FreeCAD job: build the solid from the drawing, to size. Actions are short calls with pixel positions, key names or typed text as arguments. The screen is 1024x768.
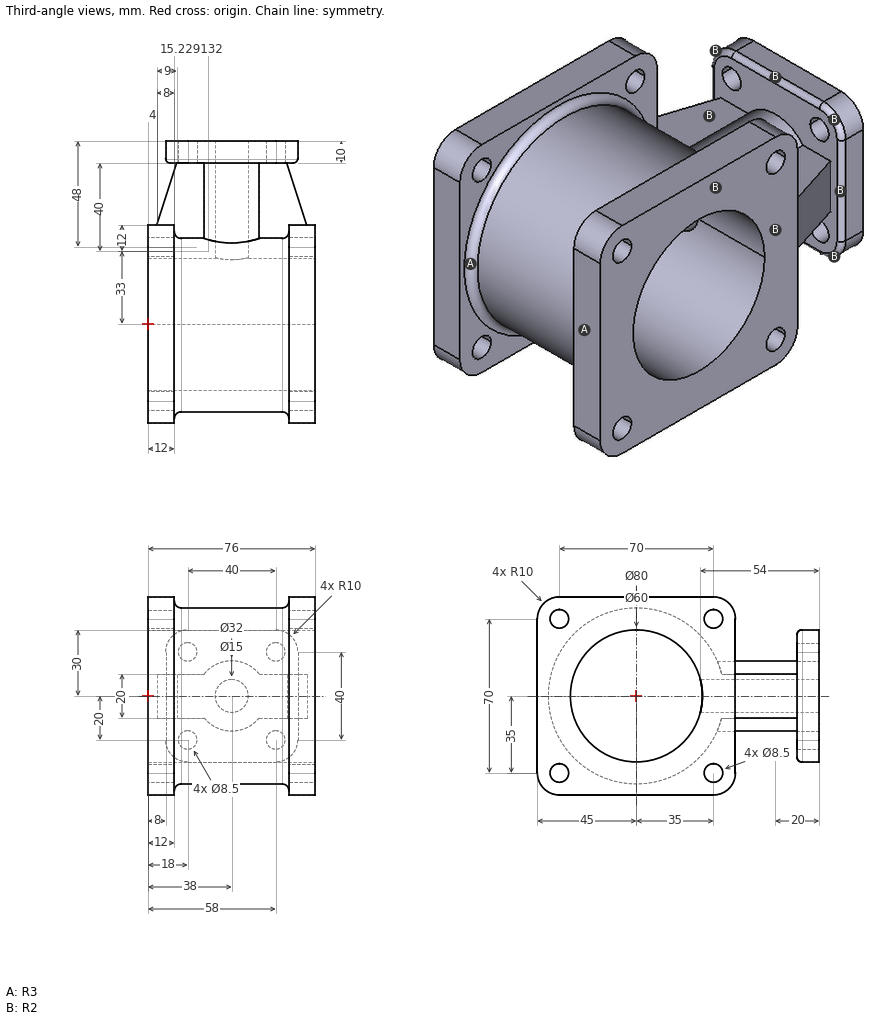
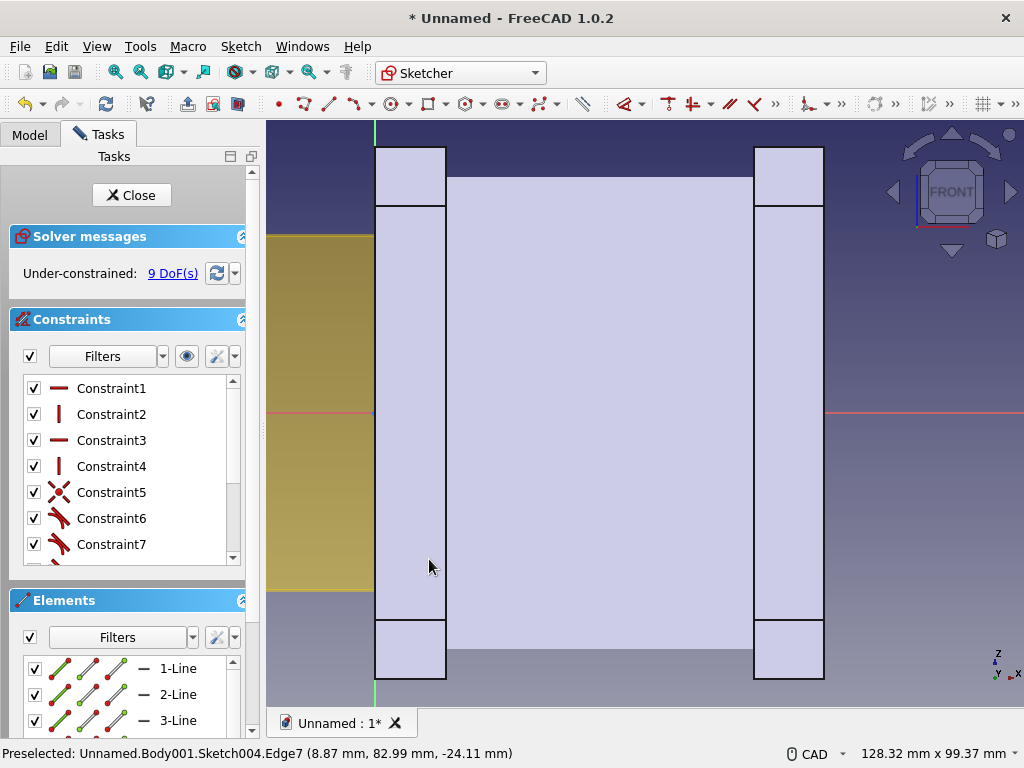
click(423, 461)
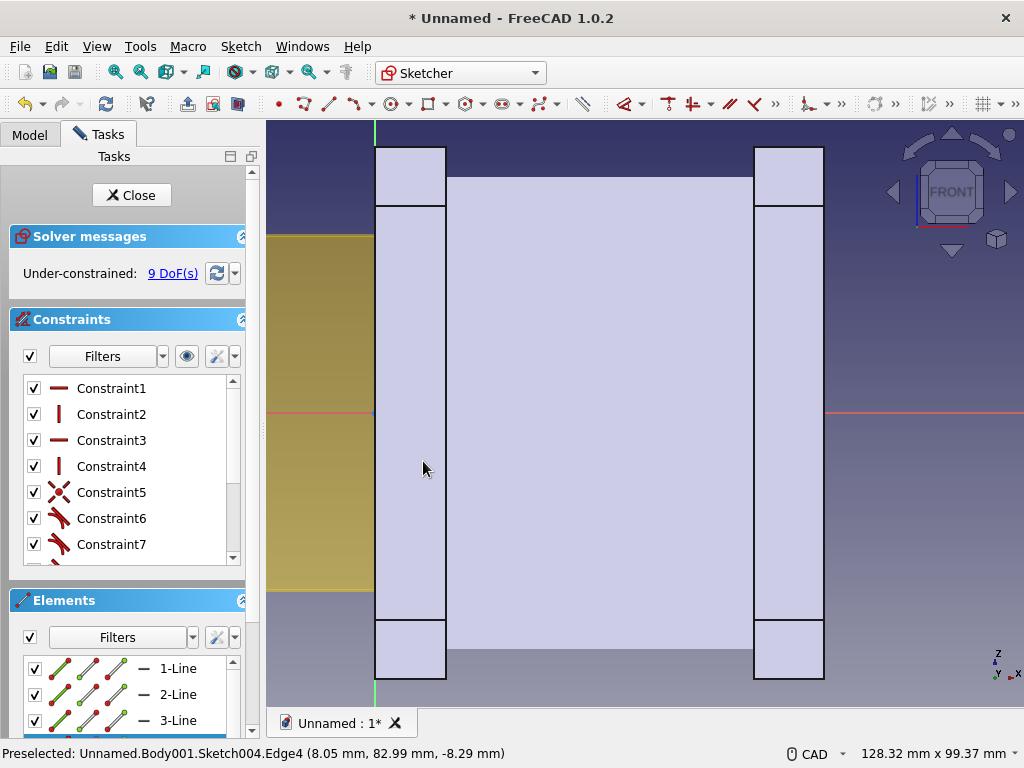
click(455, 243)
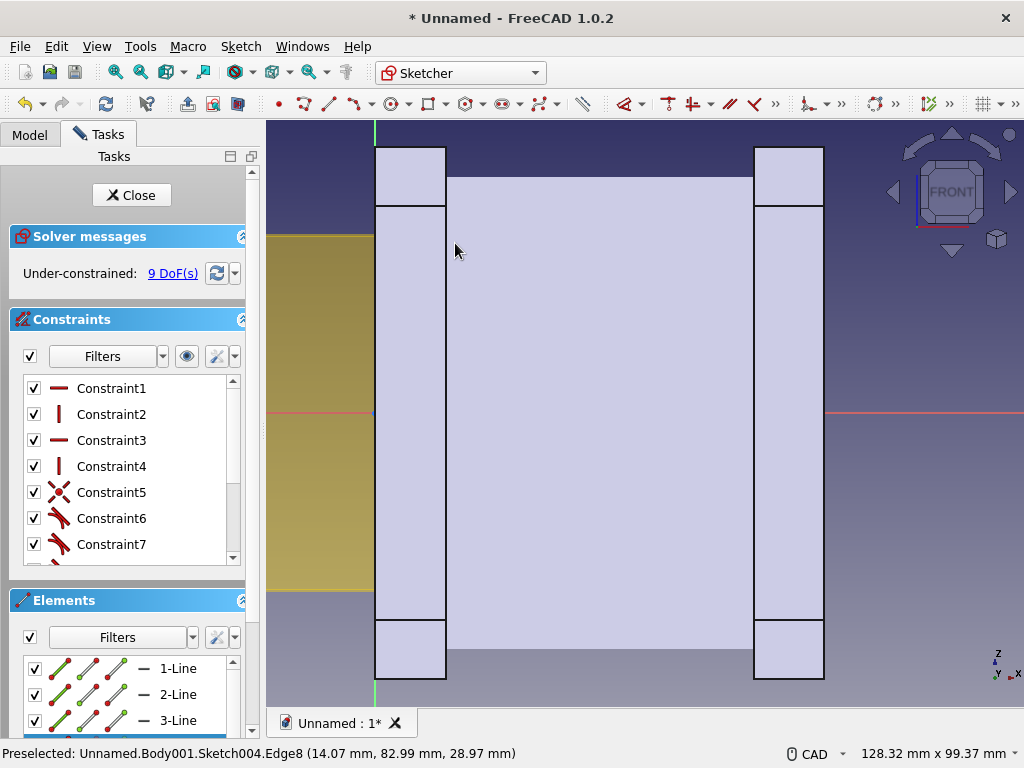
key(t)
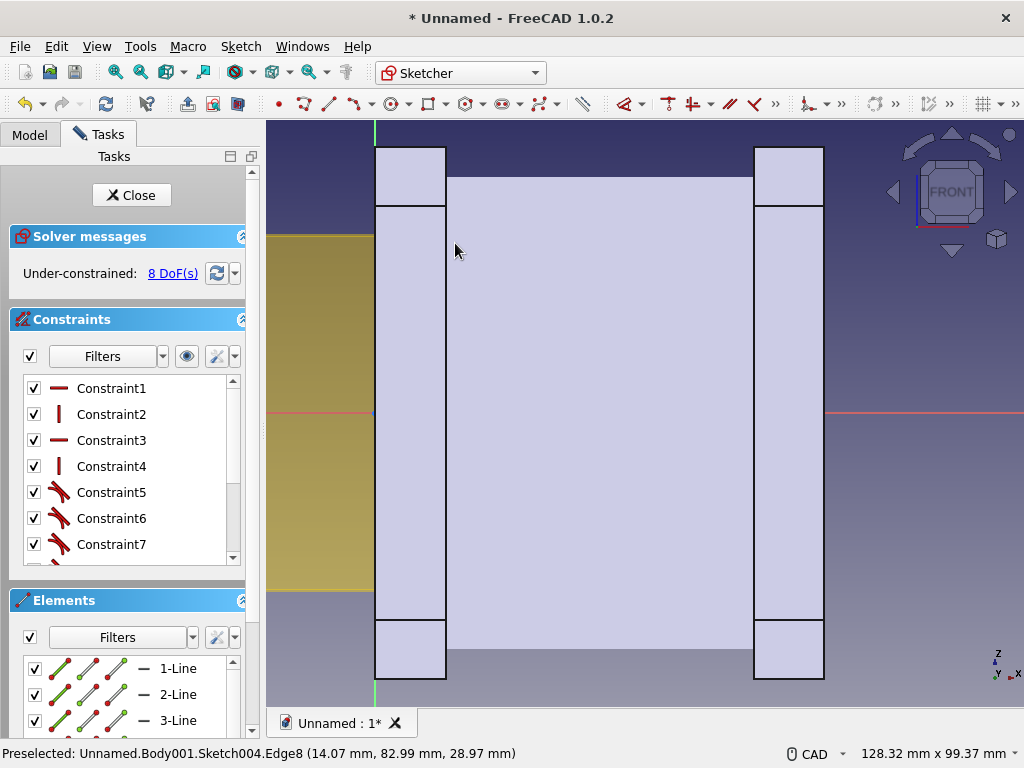
click(771, 269)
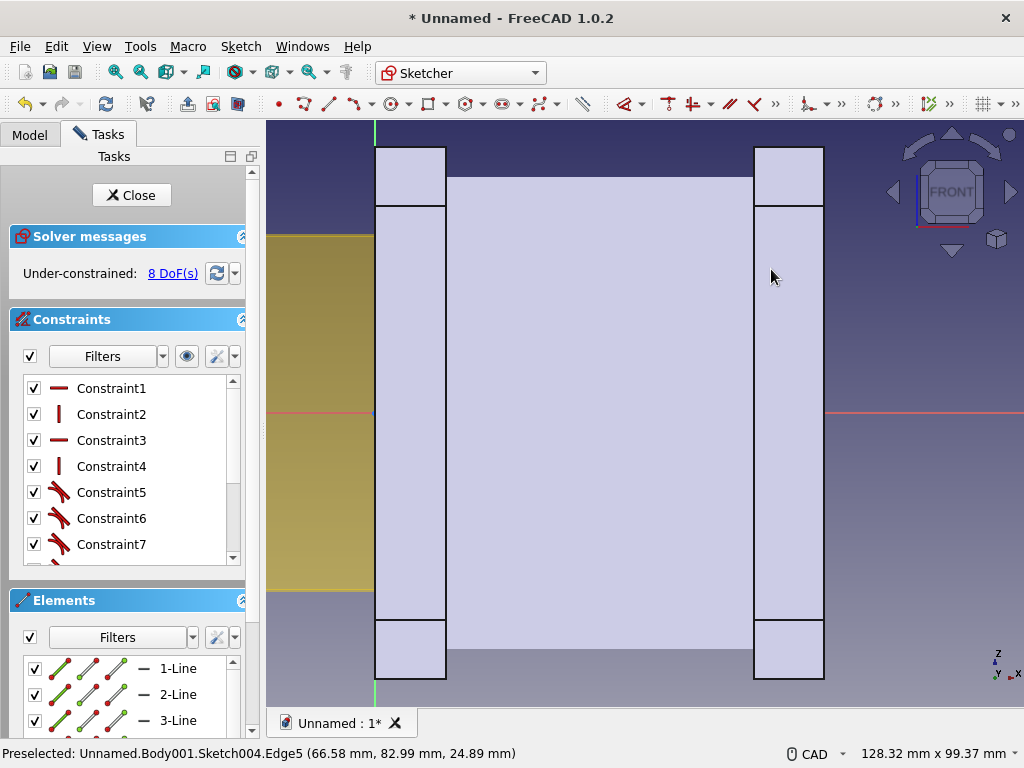
click(745, 585)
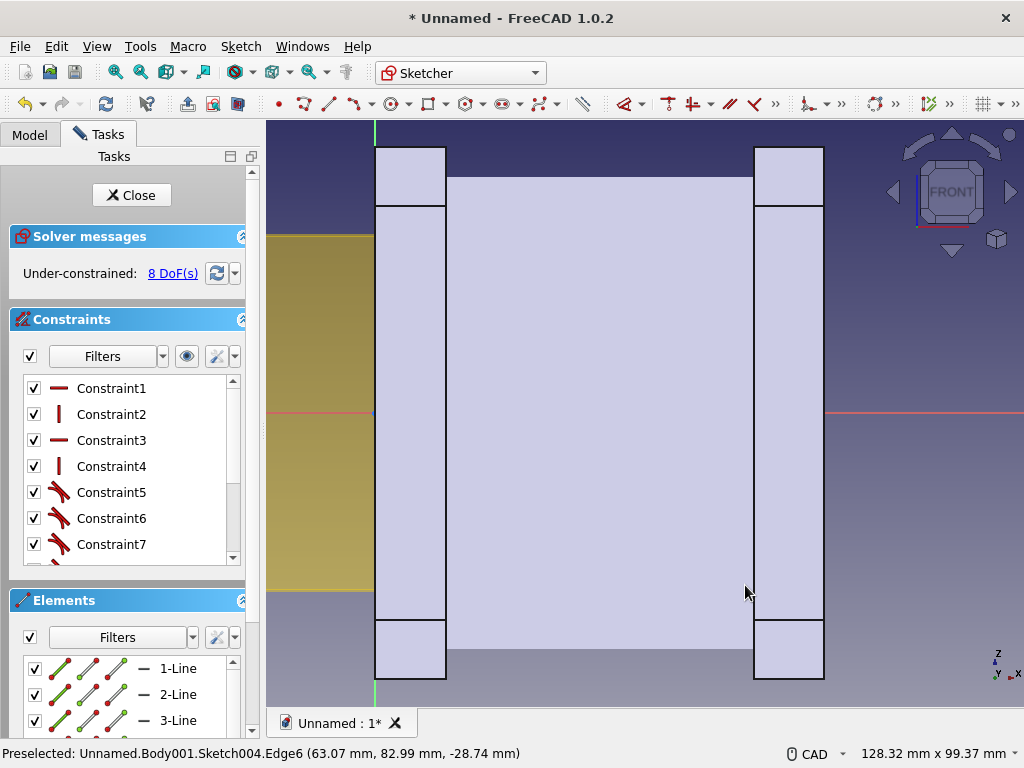
click(429, 559)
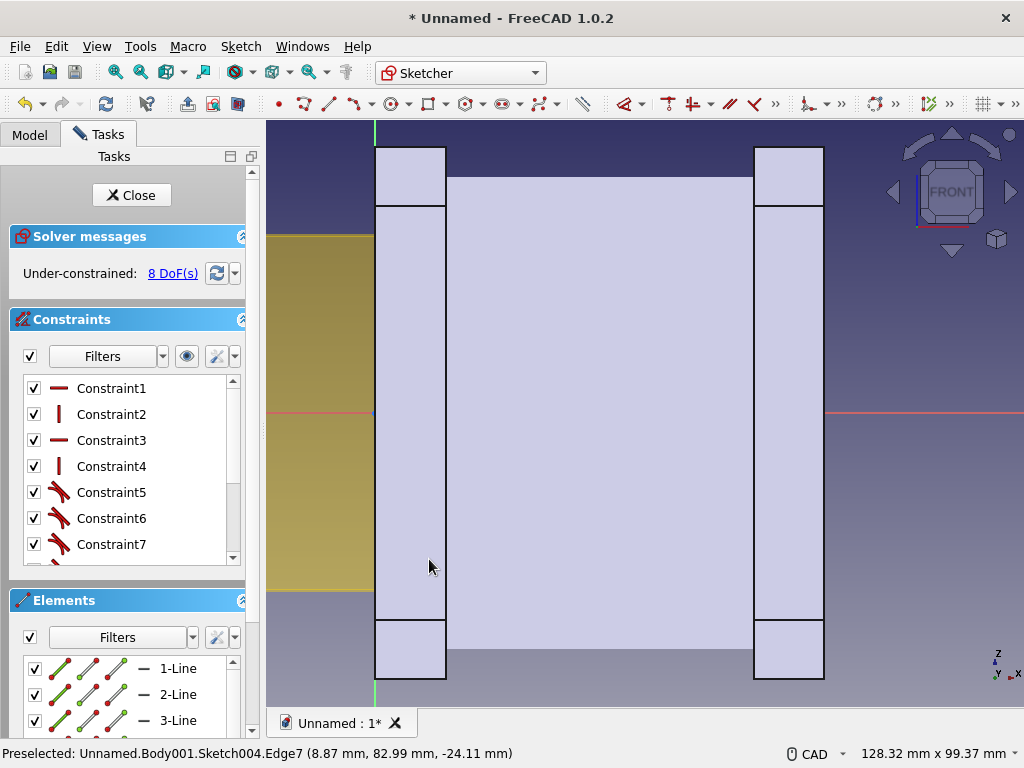
click(455, 243)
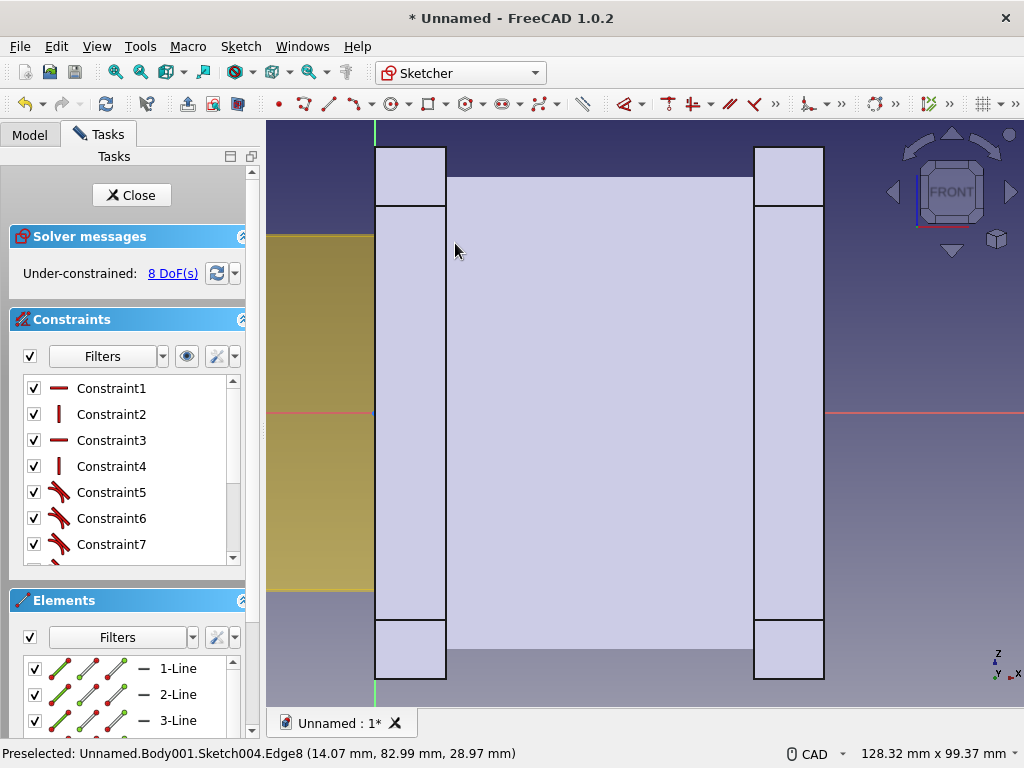
key(e)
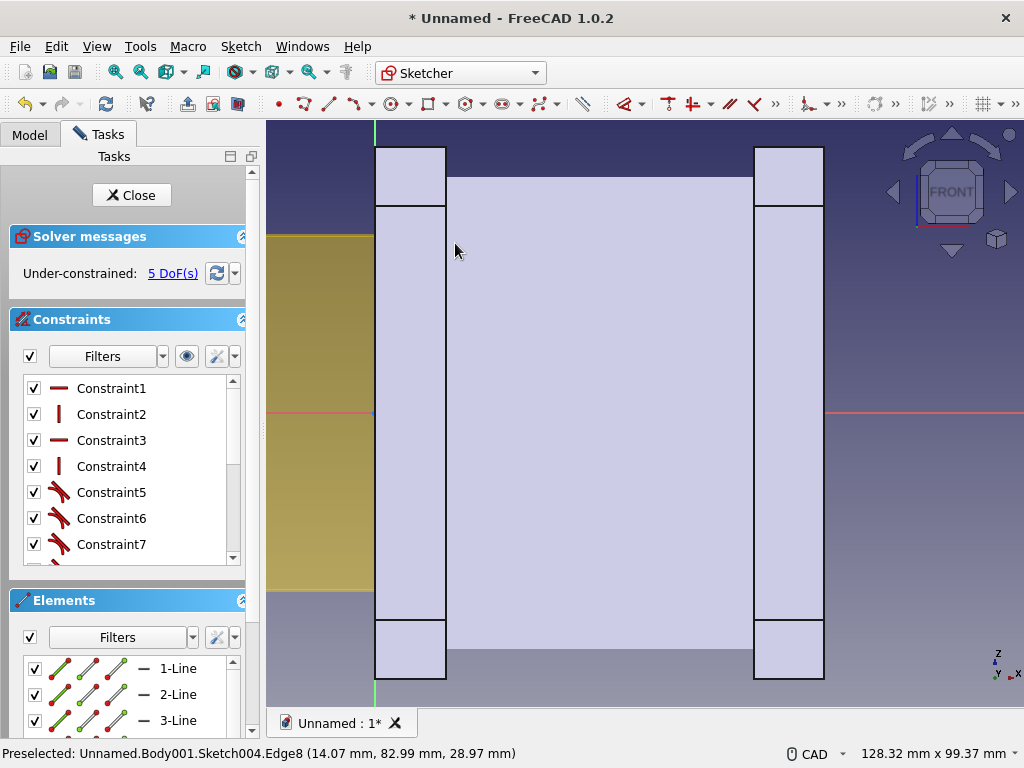
key(d)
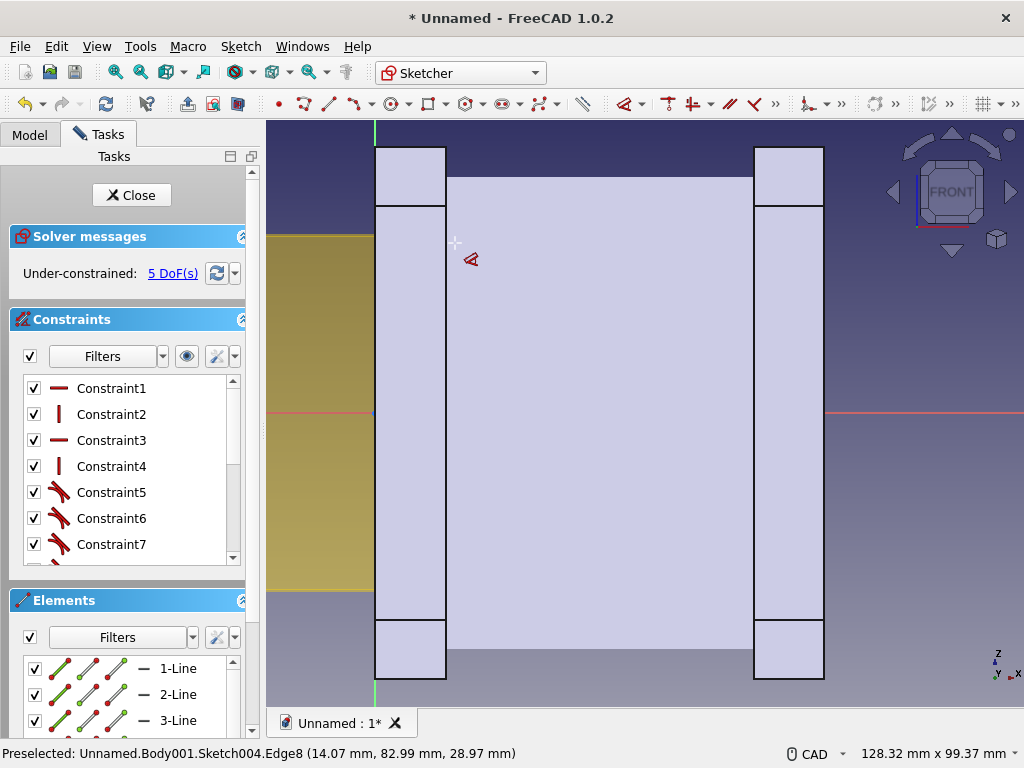
click(771, 269)
click(800, 254)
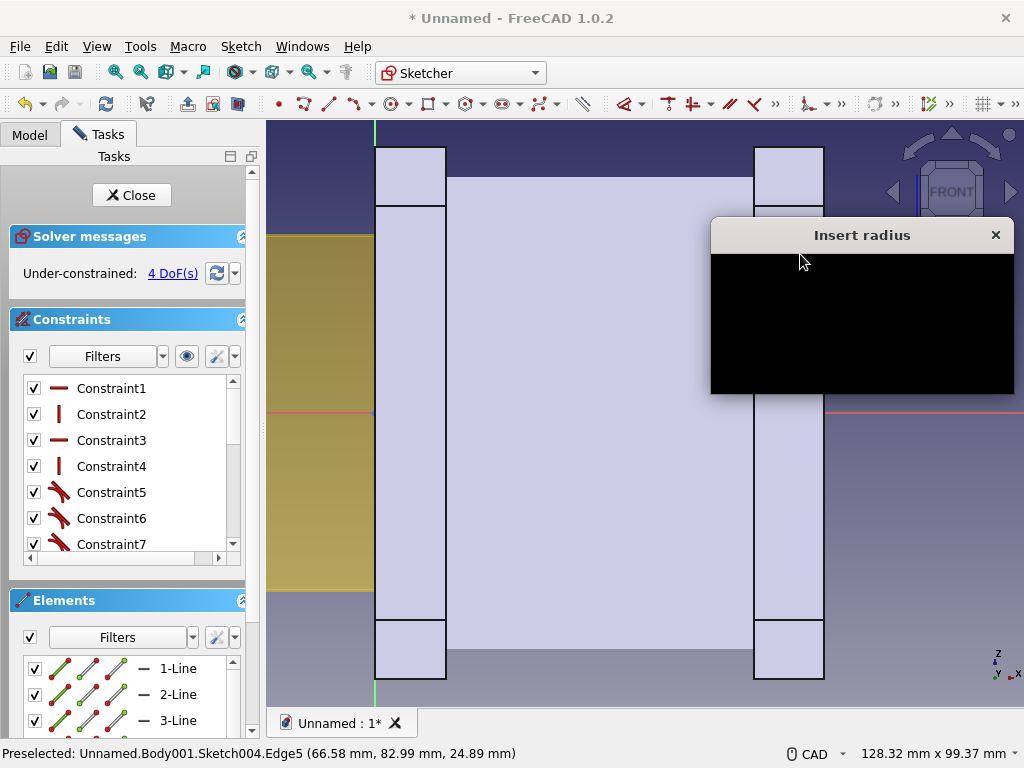
text(10)
key(Return)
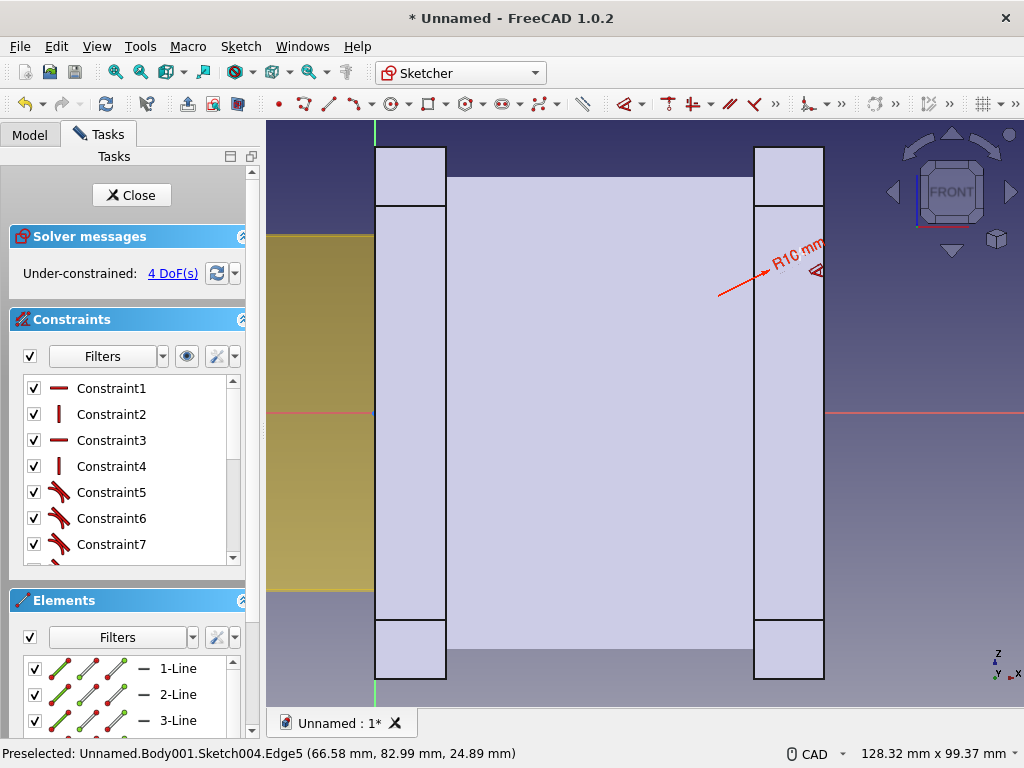
click(553, 237)
click(600, 203)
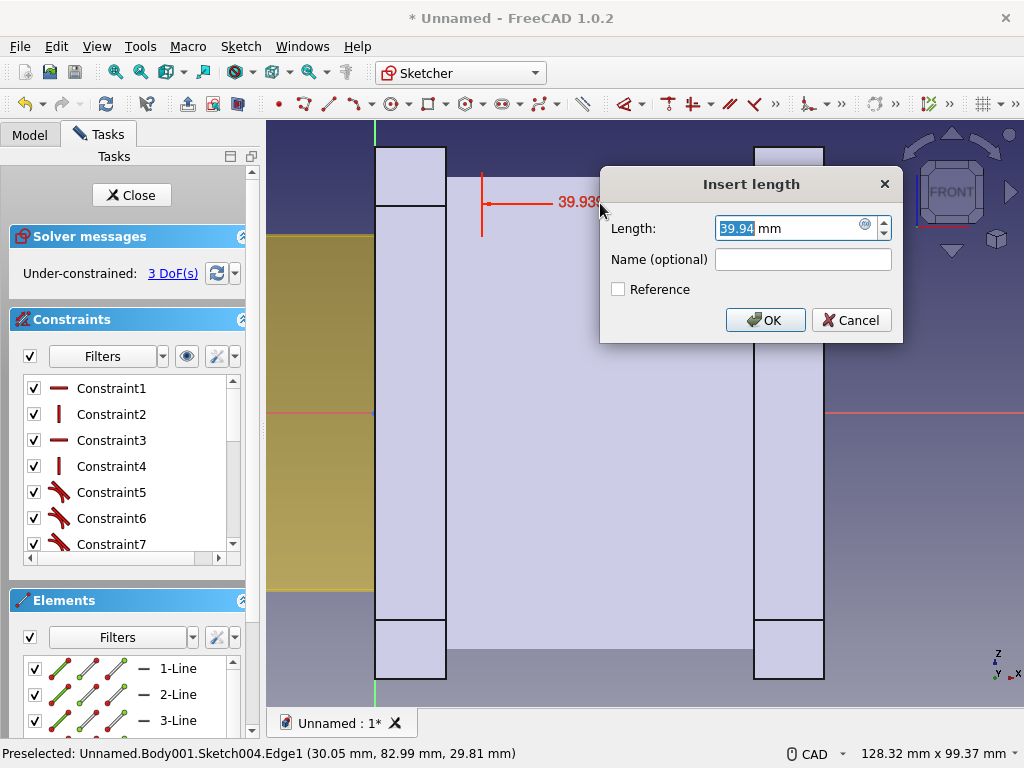
text(40)
key(Return)